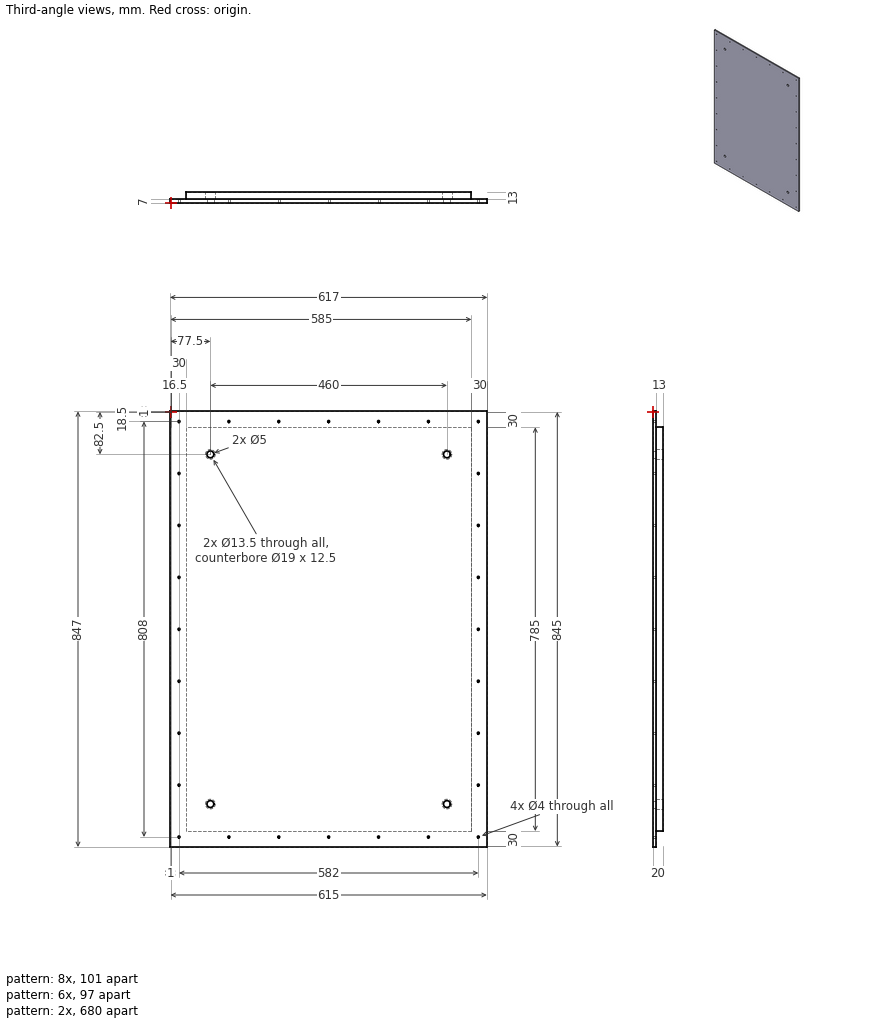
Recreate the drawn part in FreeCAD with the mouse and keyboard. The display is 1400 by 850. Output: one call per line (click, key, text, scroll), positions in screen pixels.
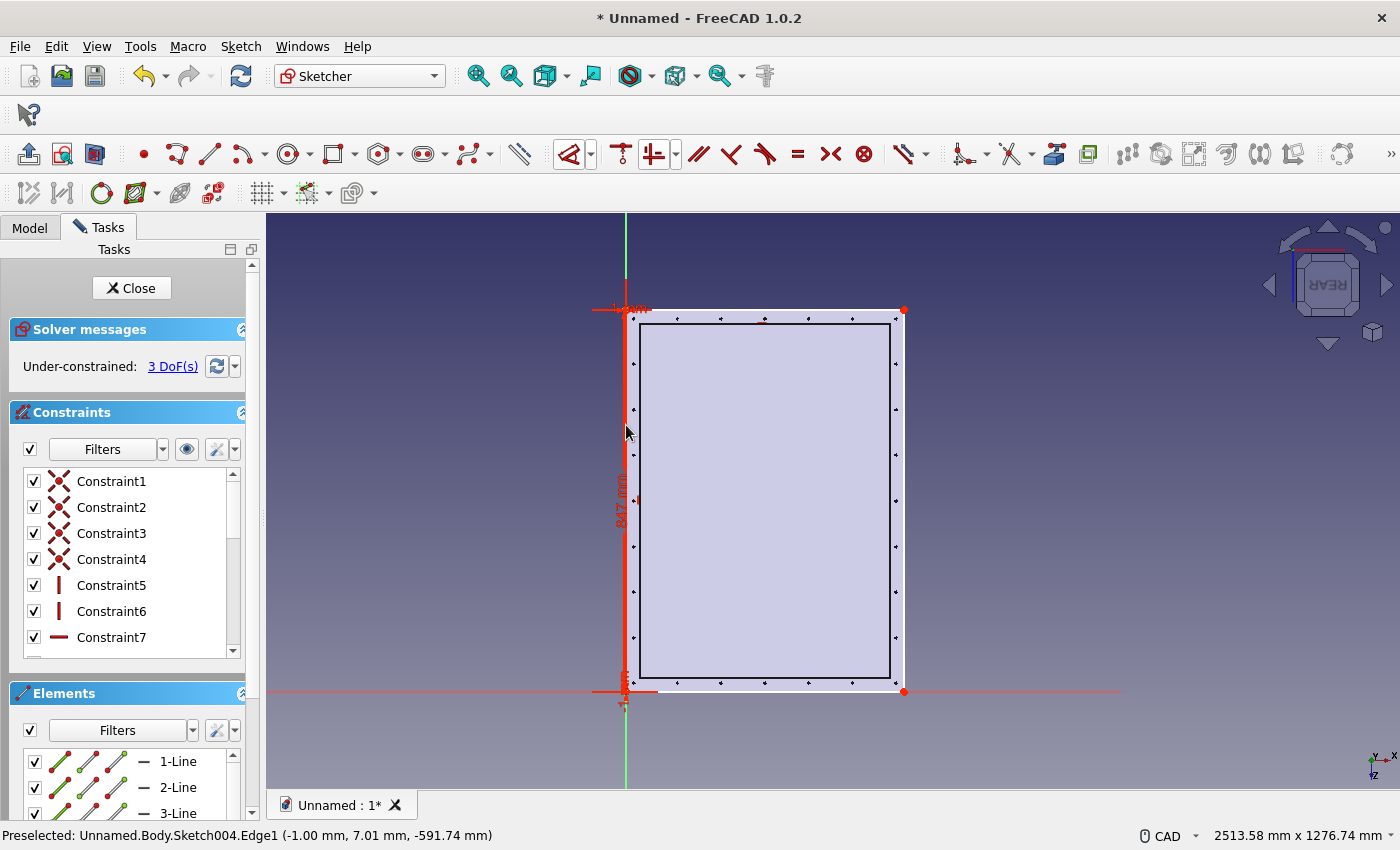
scroll(709, 692, up, 15)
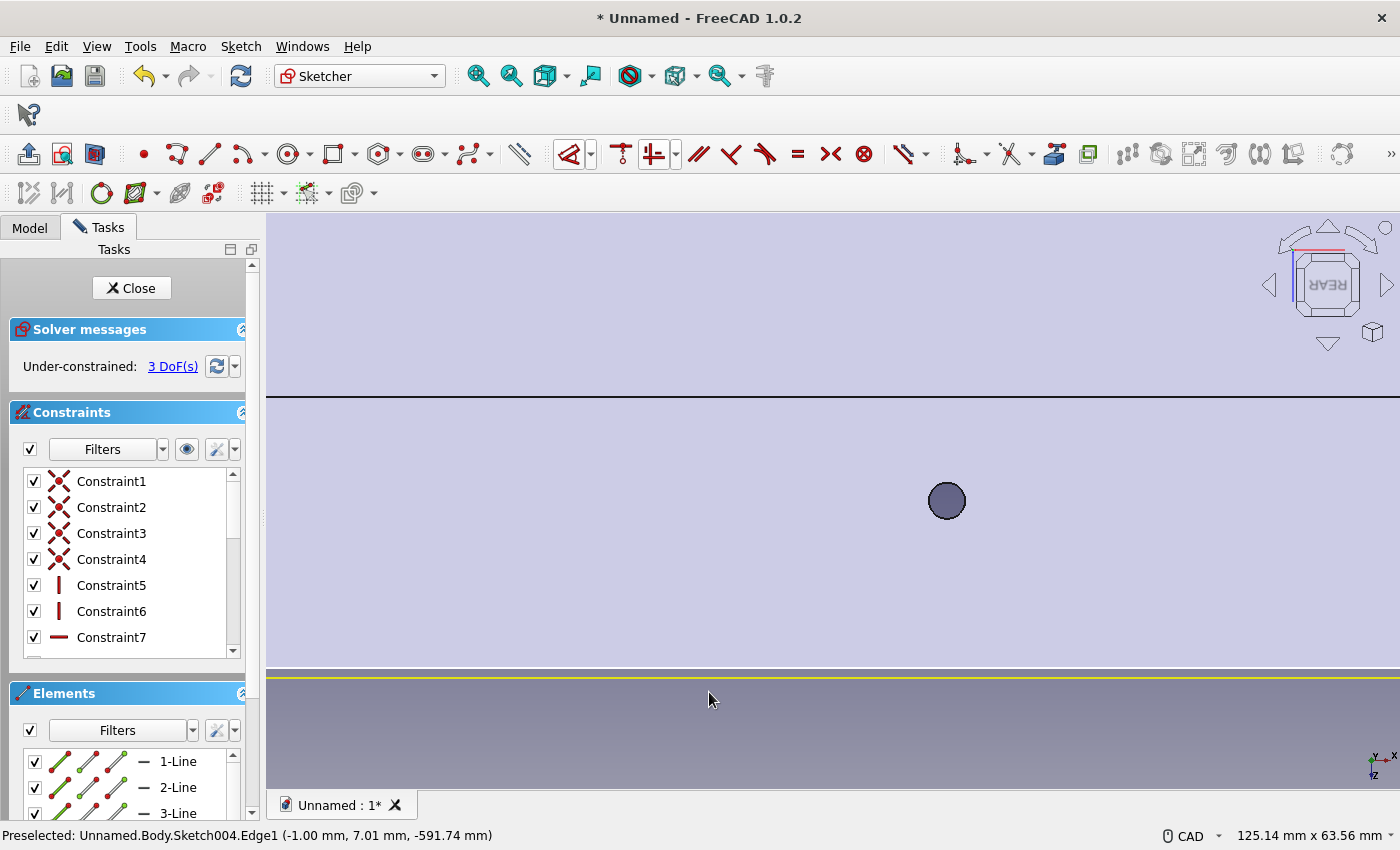
click(708, 678)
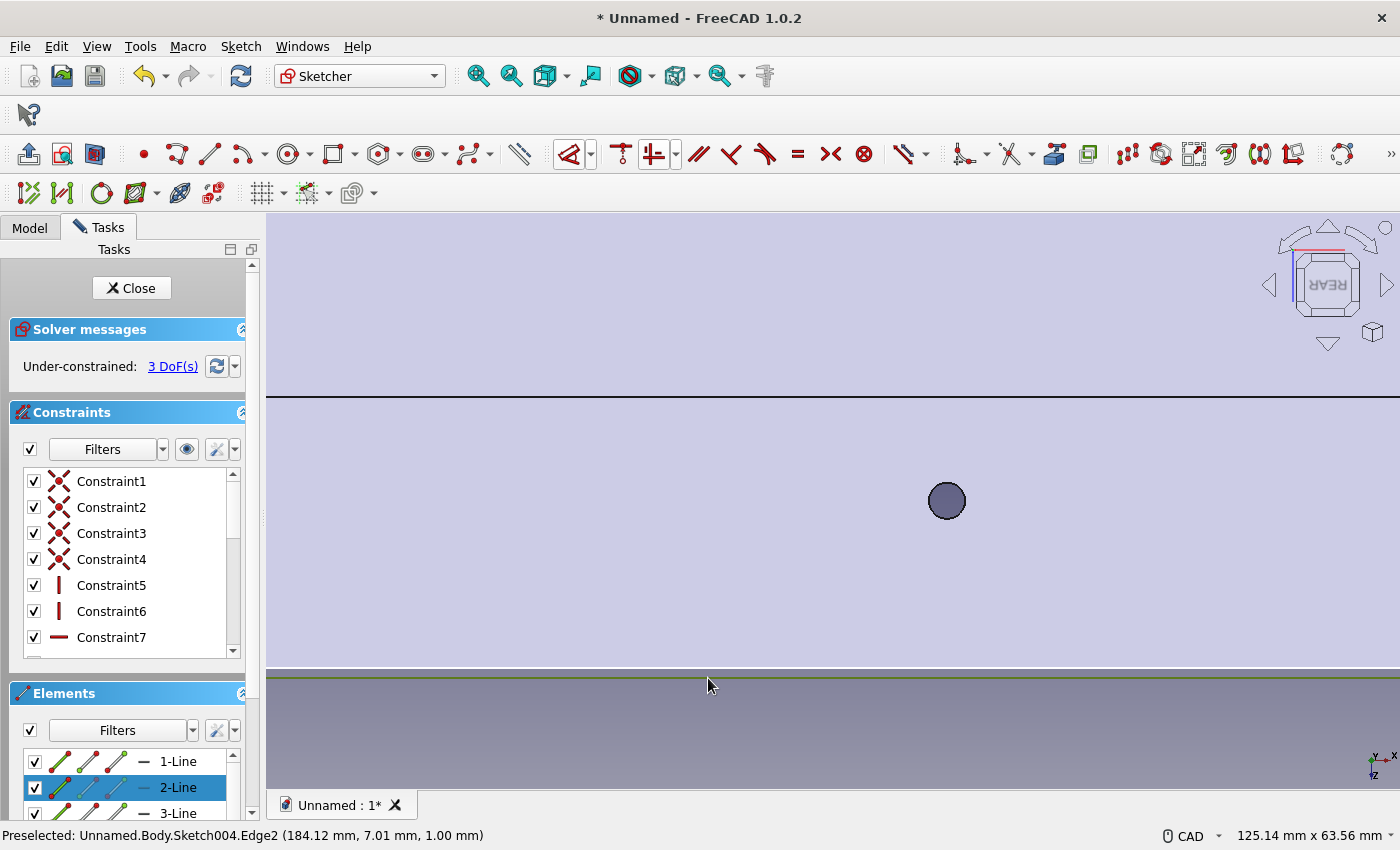
key(l)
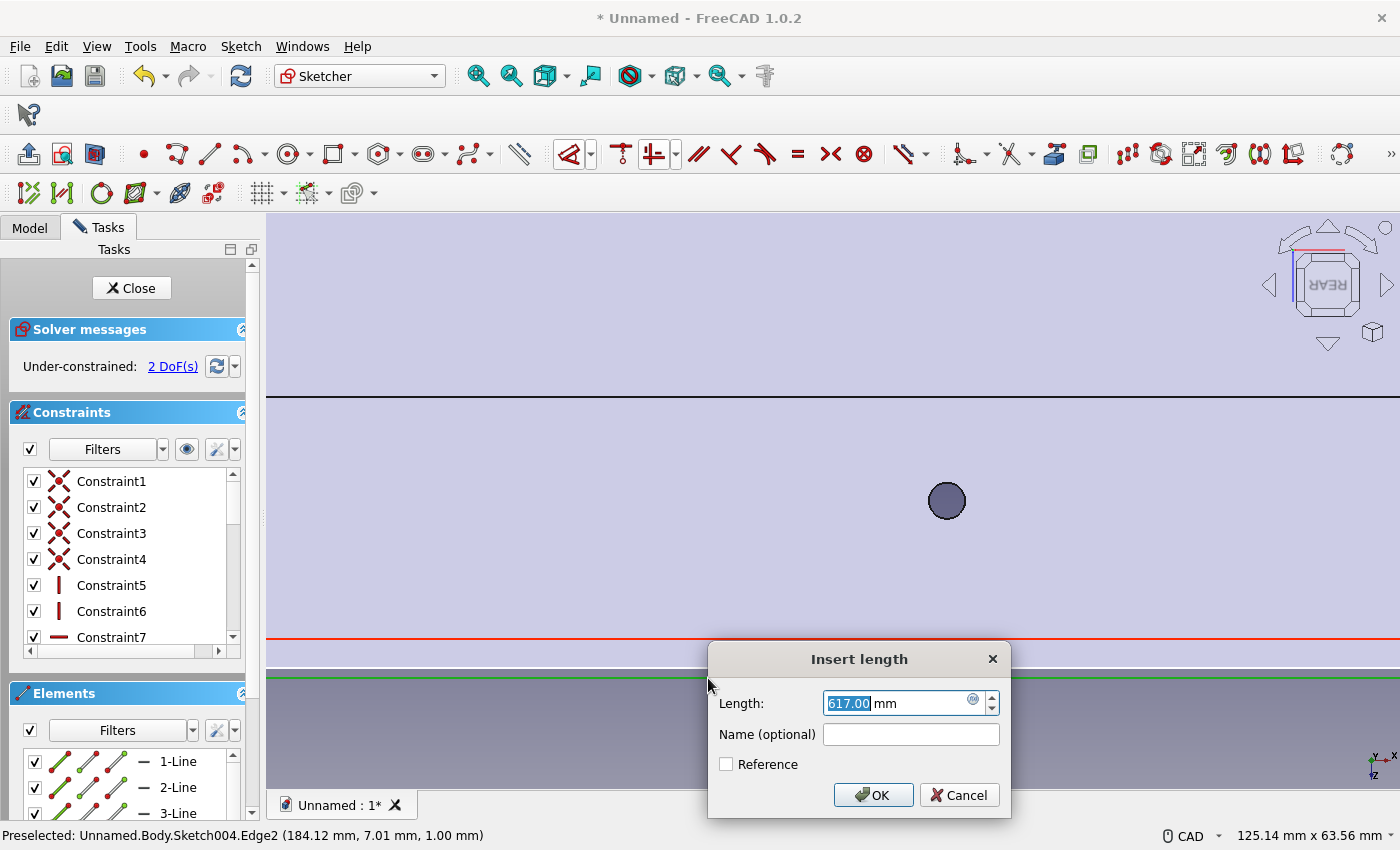
text(617)
key(Return)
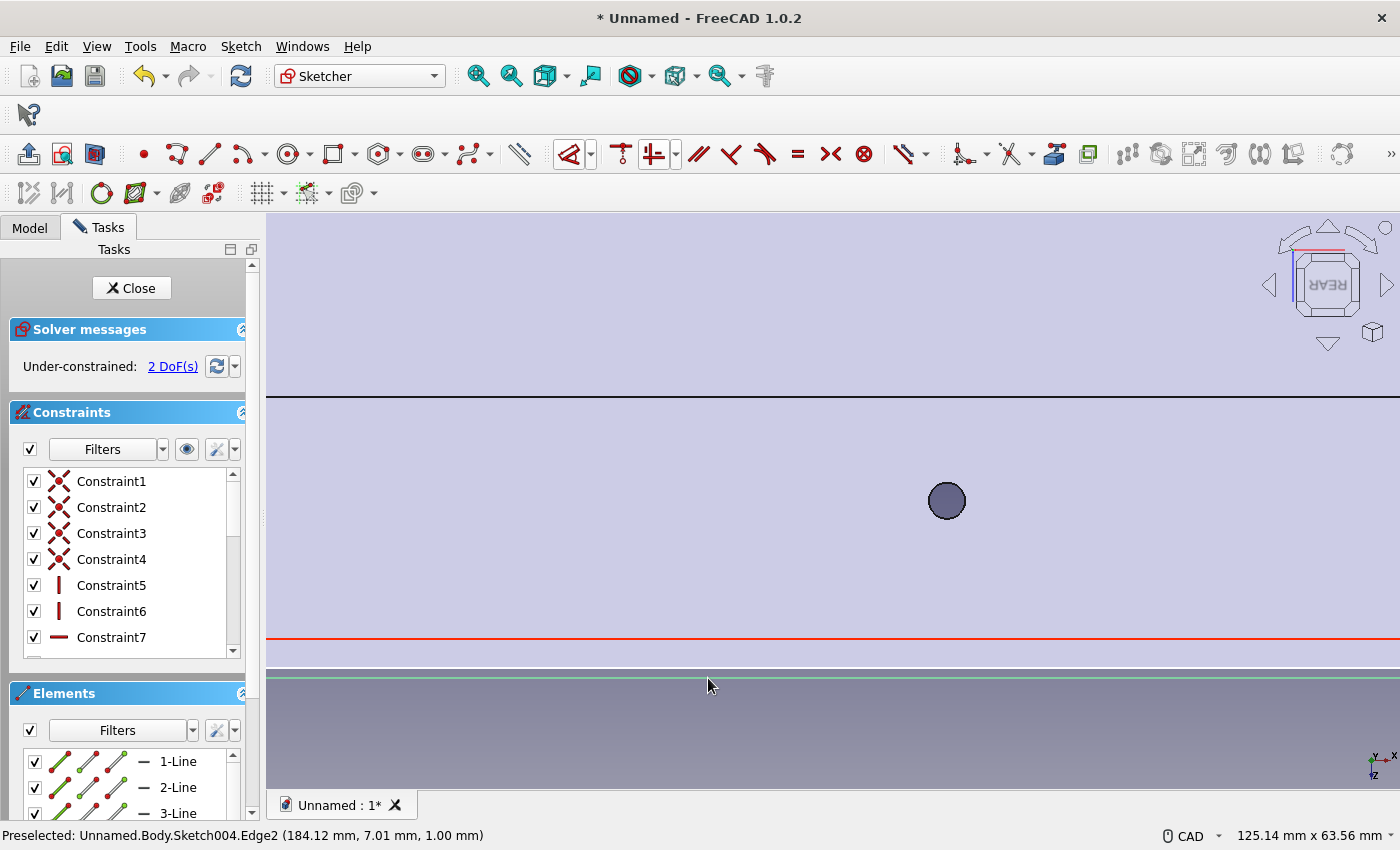
click(711, 668)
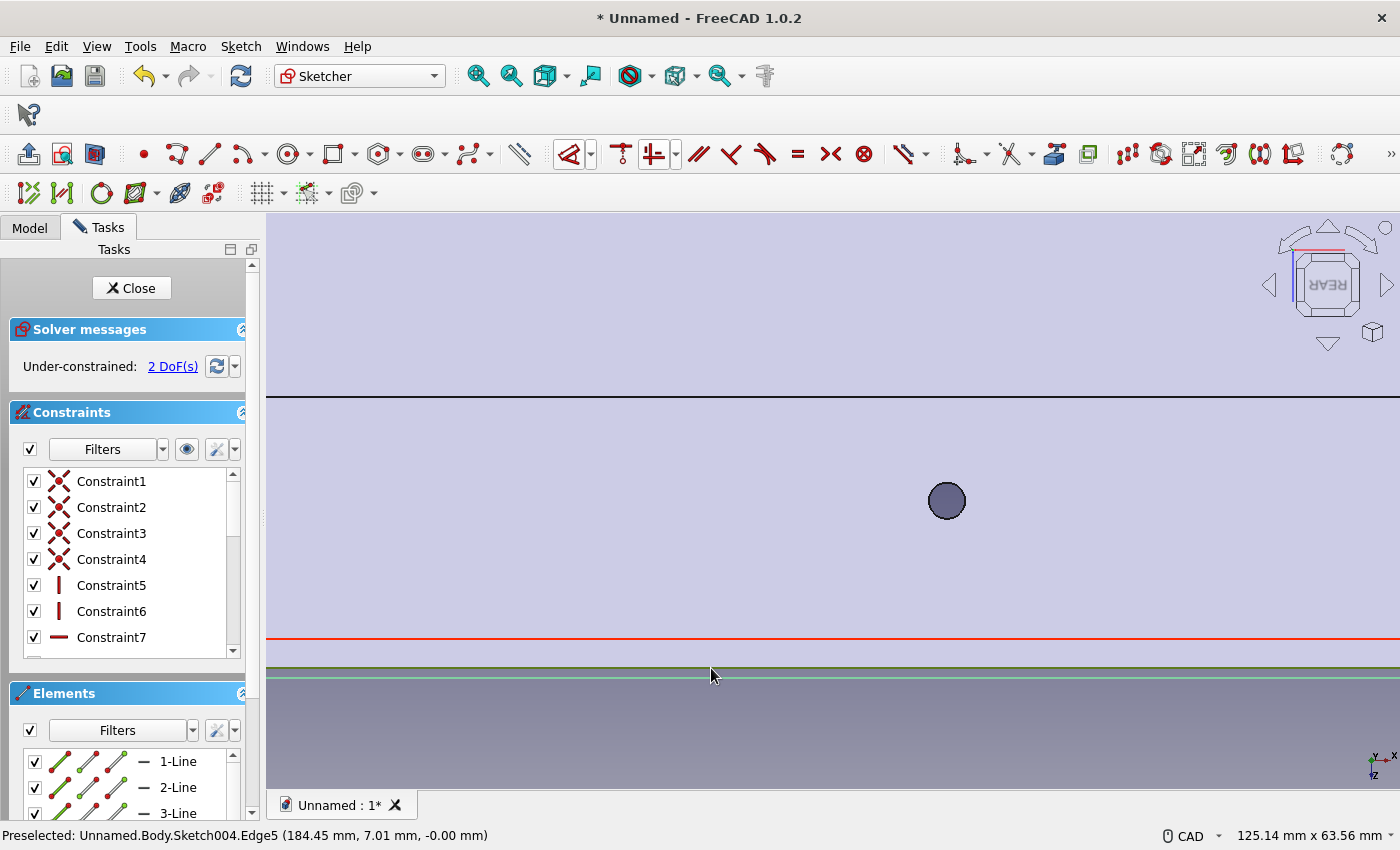
key(l)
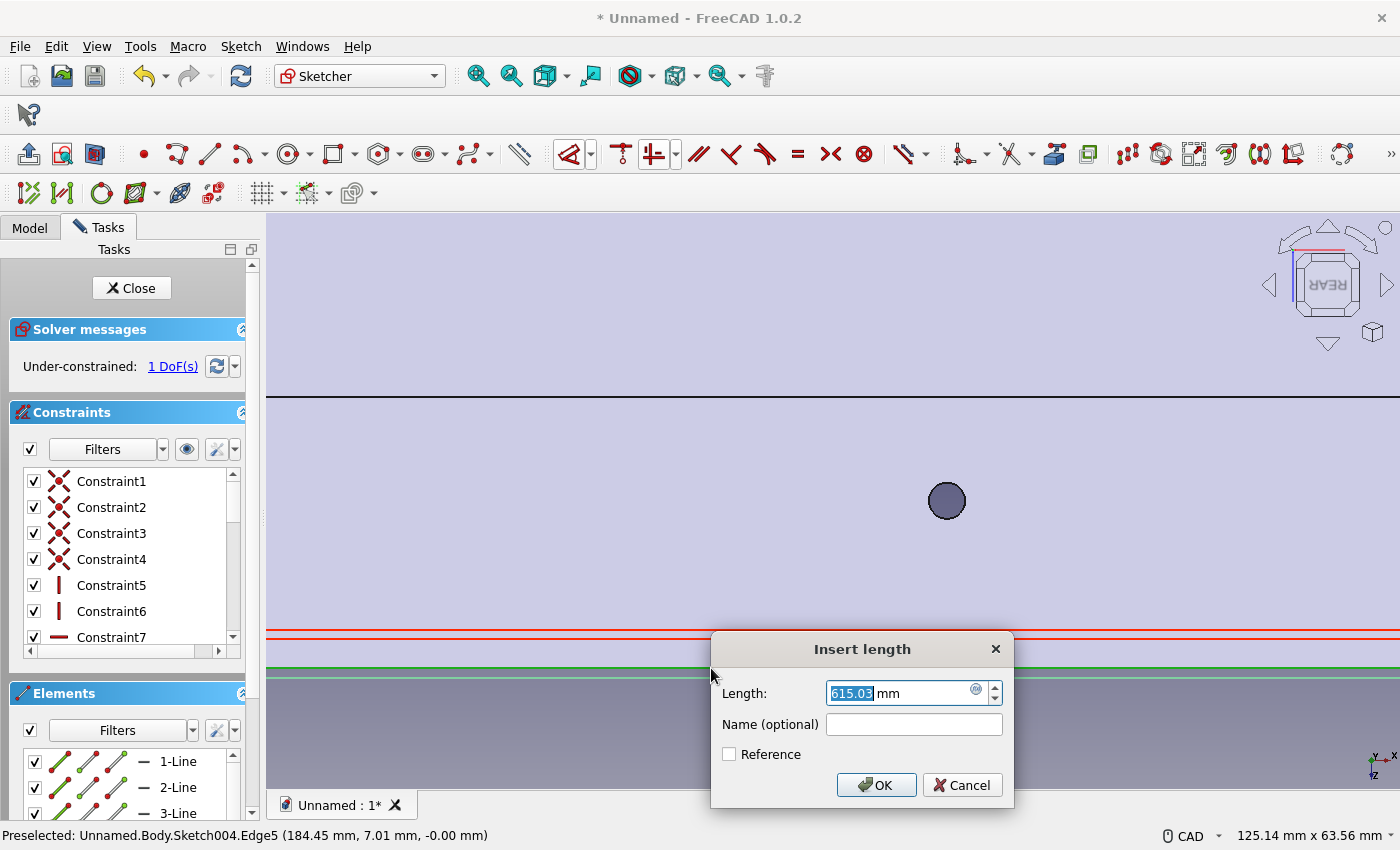
text(615)
key(Return)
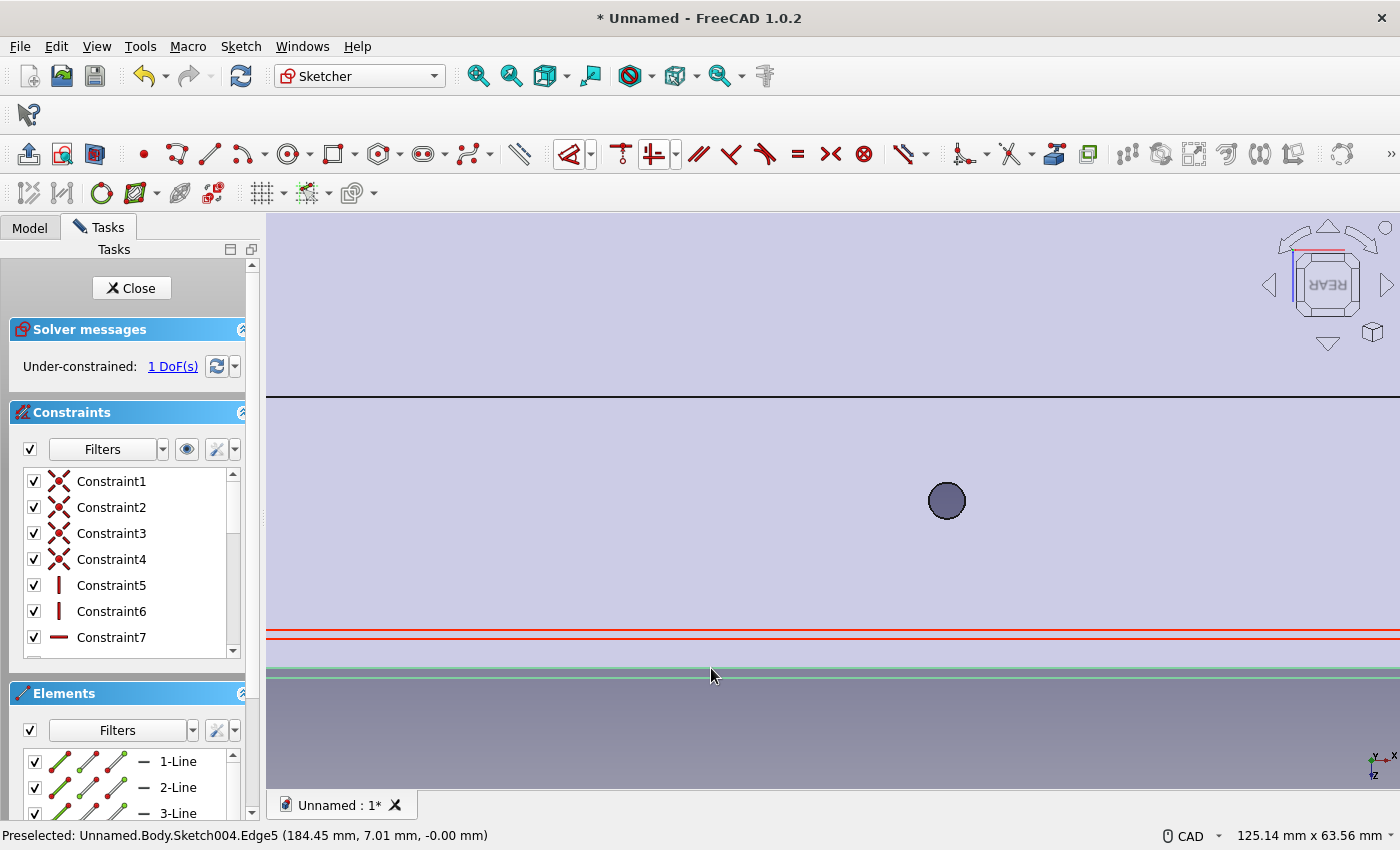
scroll(709, 693, down, 15)